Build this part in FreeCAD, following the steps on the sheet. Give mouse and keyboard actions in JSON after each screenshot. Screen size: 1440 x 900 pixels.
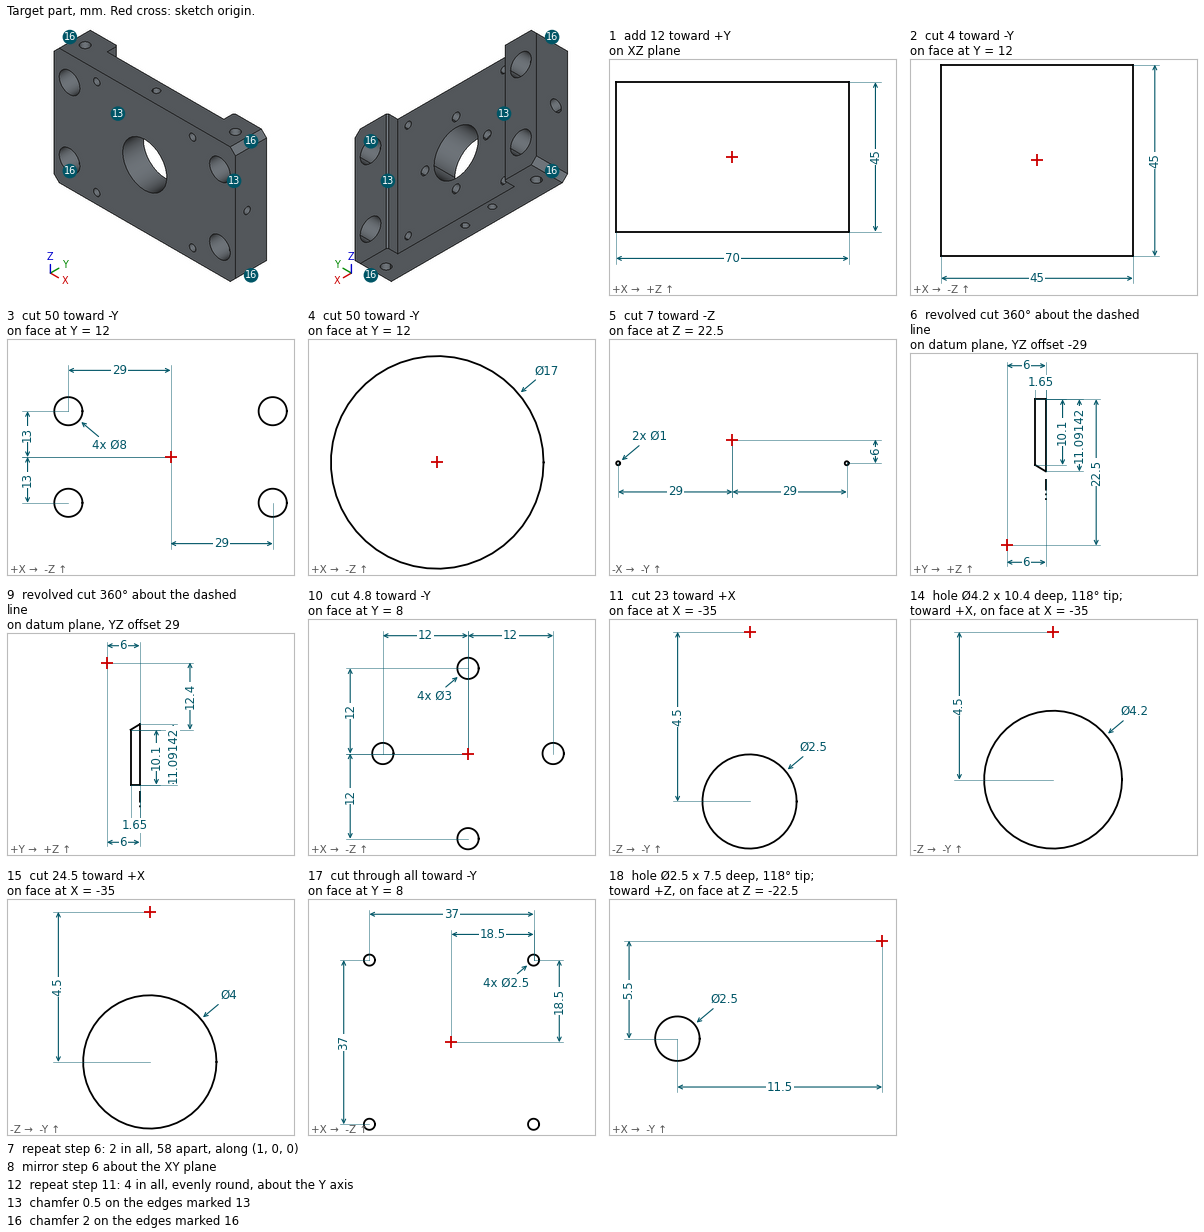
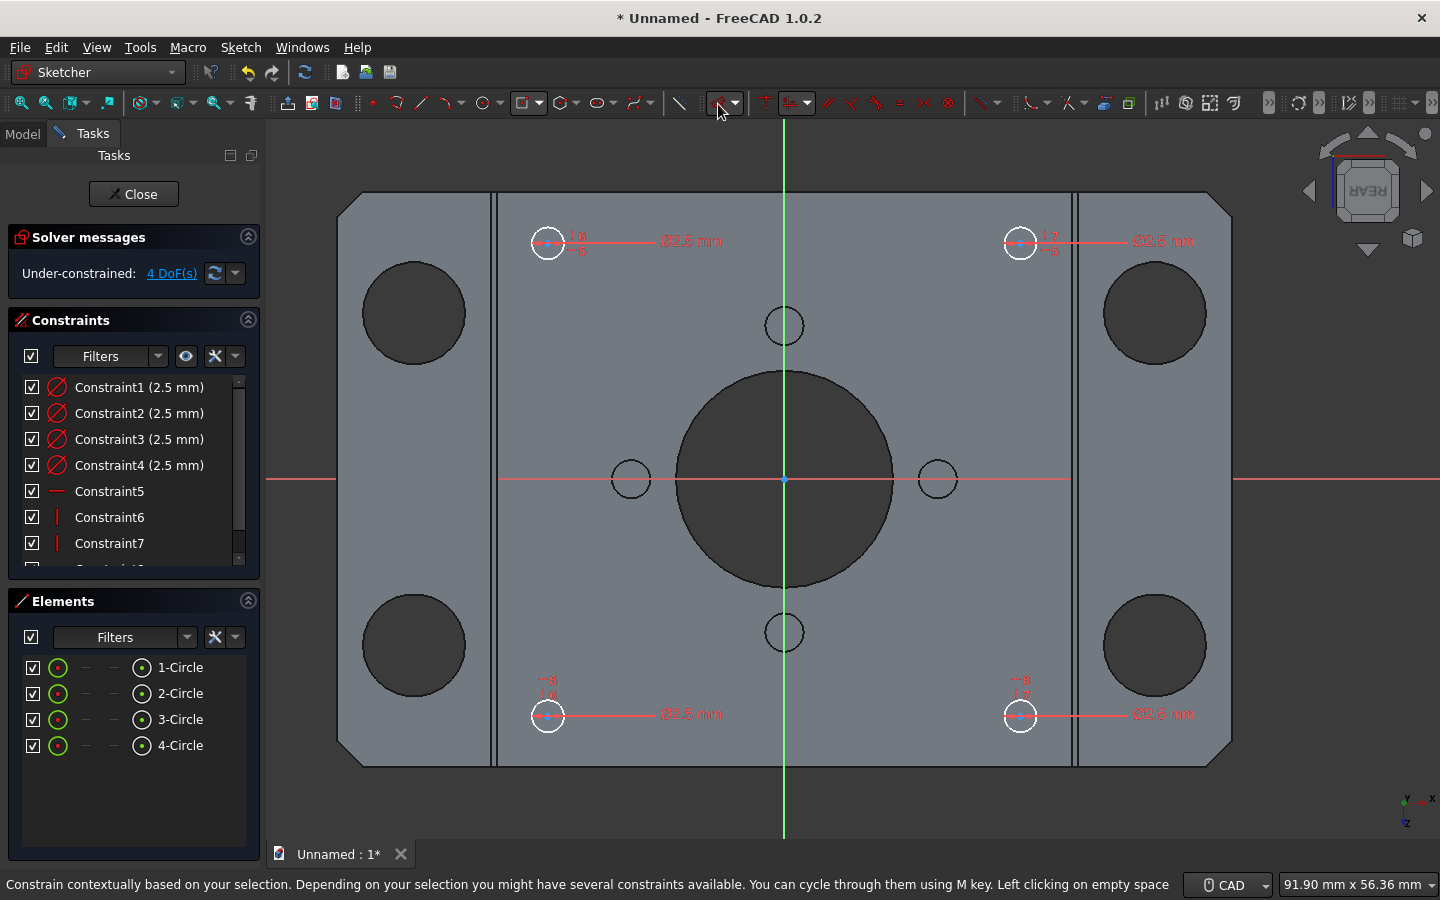
{"action": "left_click", "coordinate": [1021, 243]}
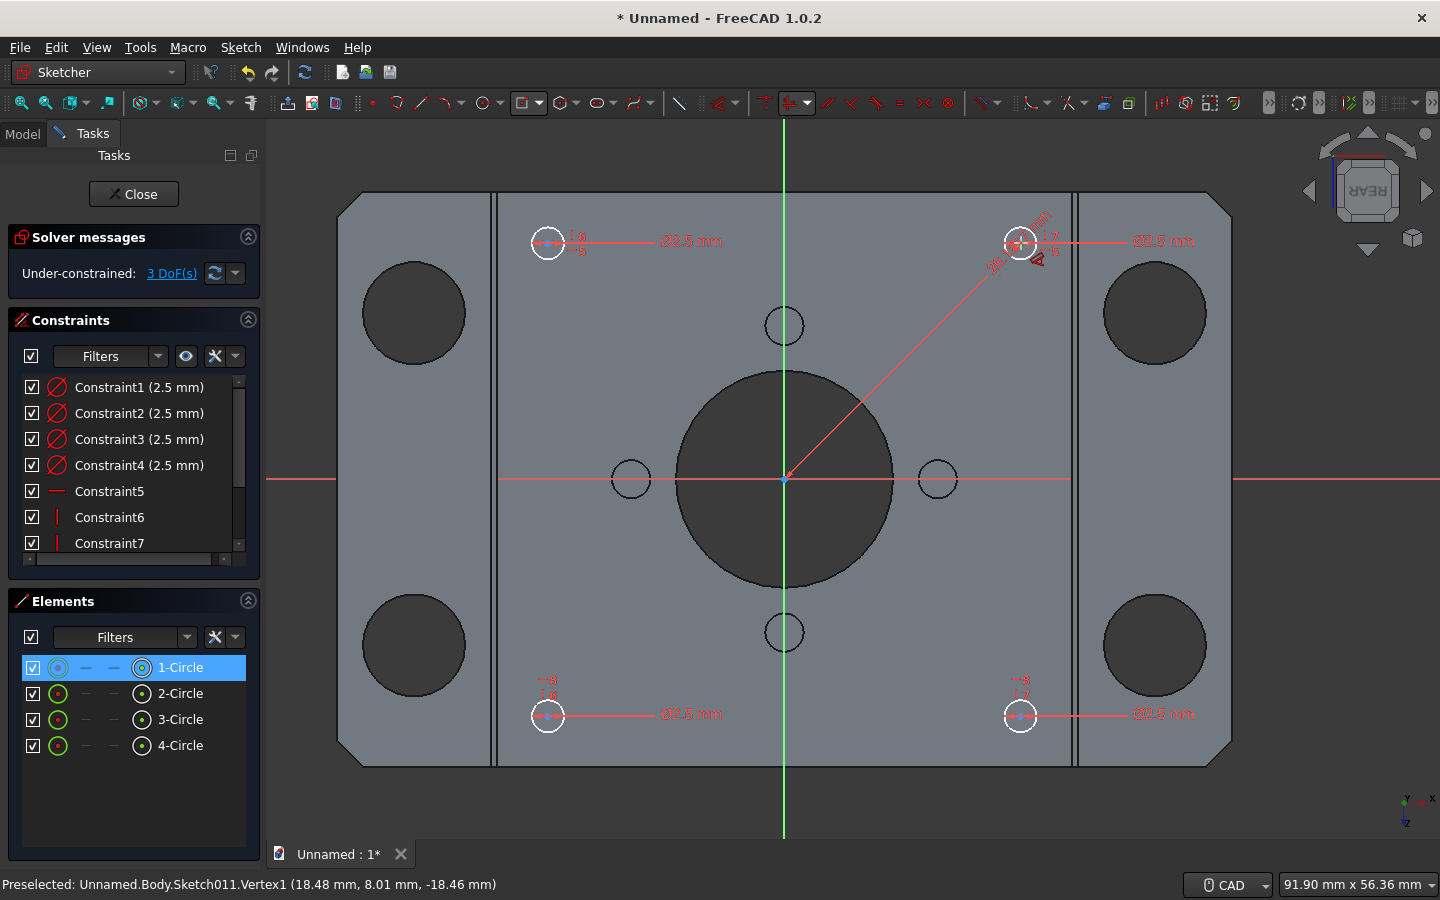
{"action": "left_click", "coordinate": [548, 243]}
{"action": "left_click", "coordinate": [676, 209]}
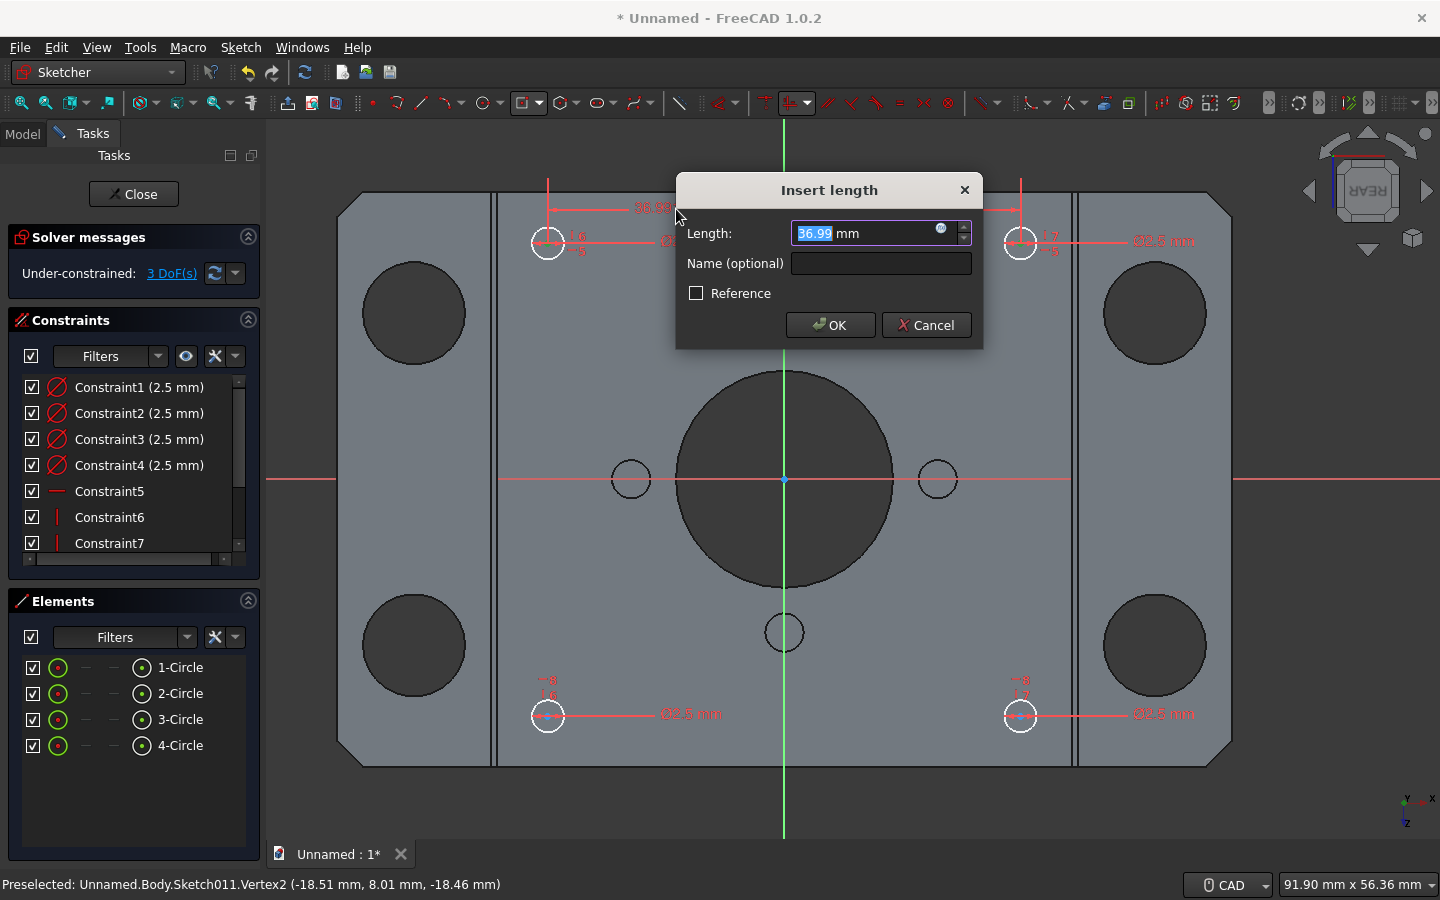
{"action": "type", "text": "37"}
{"action": "key", "text": "Return"}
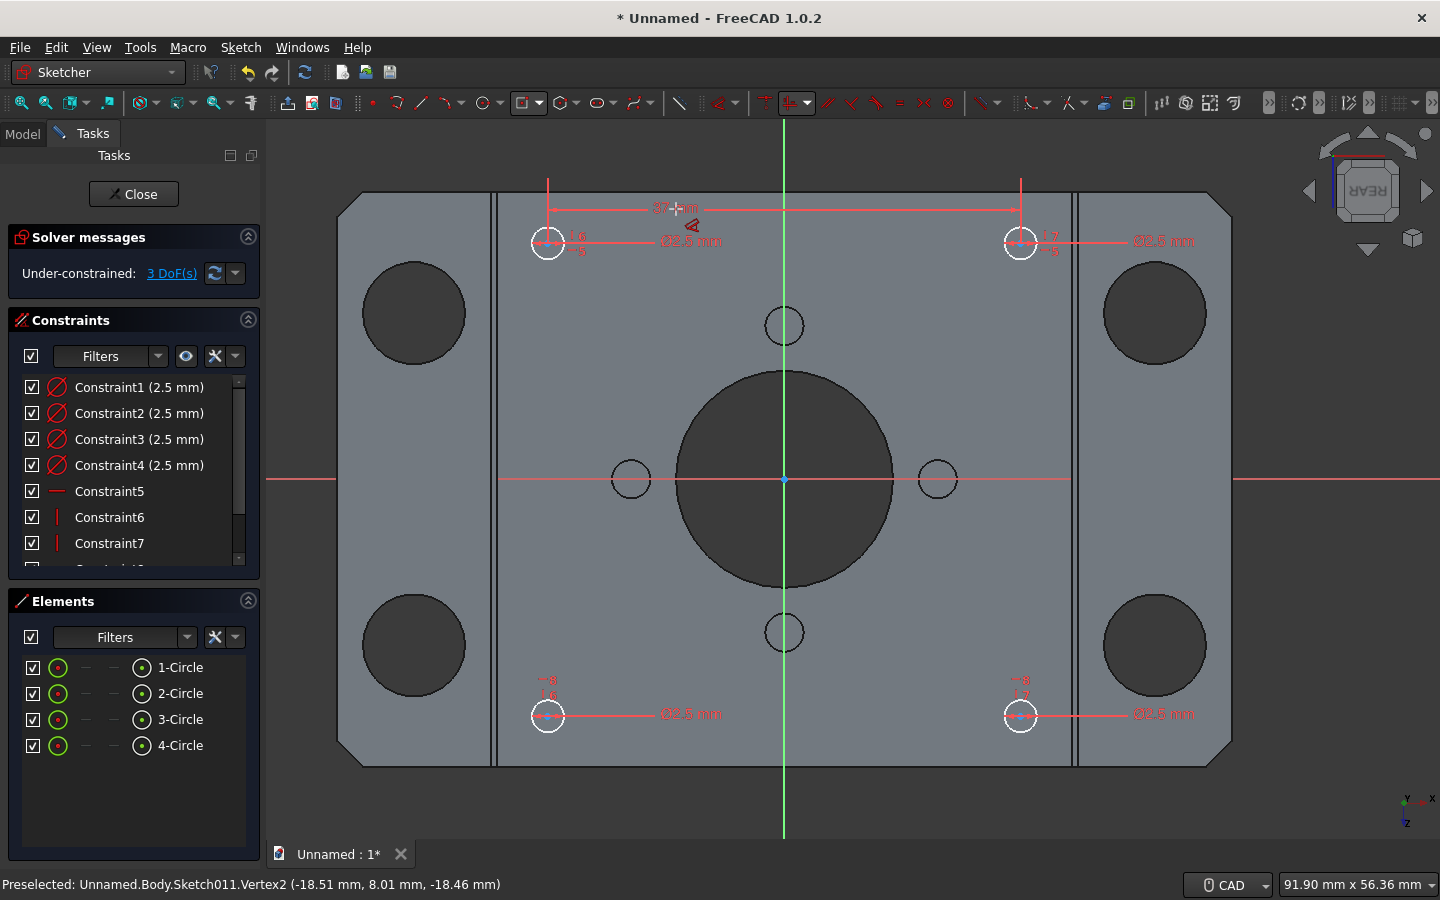
{"action": "left_click", "coordinate": [548, 243]}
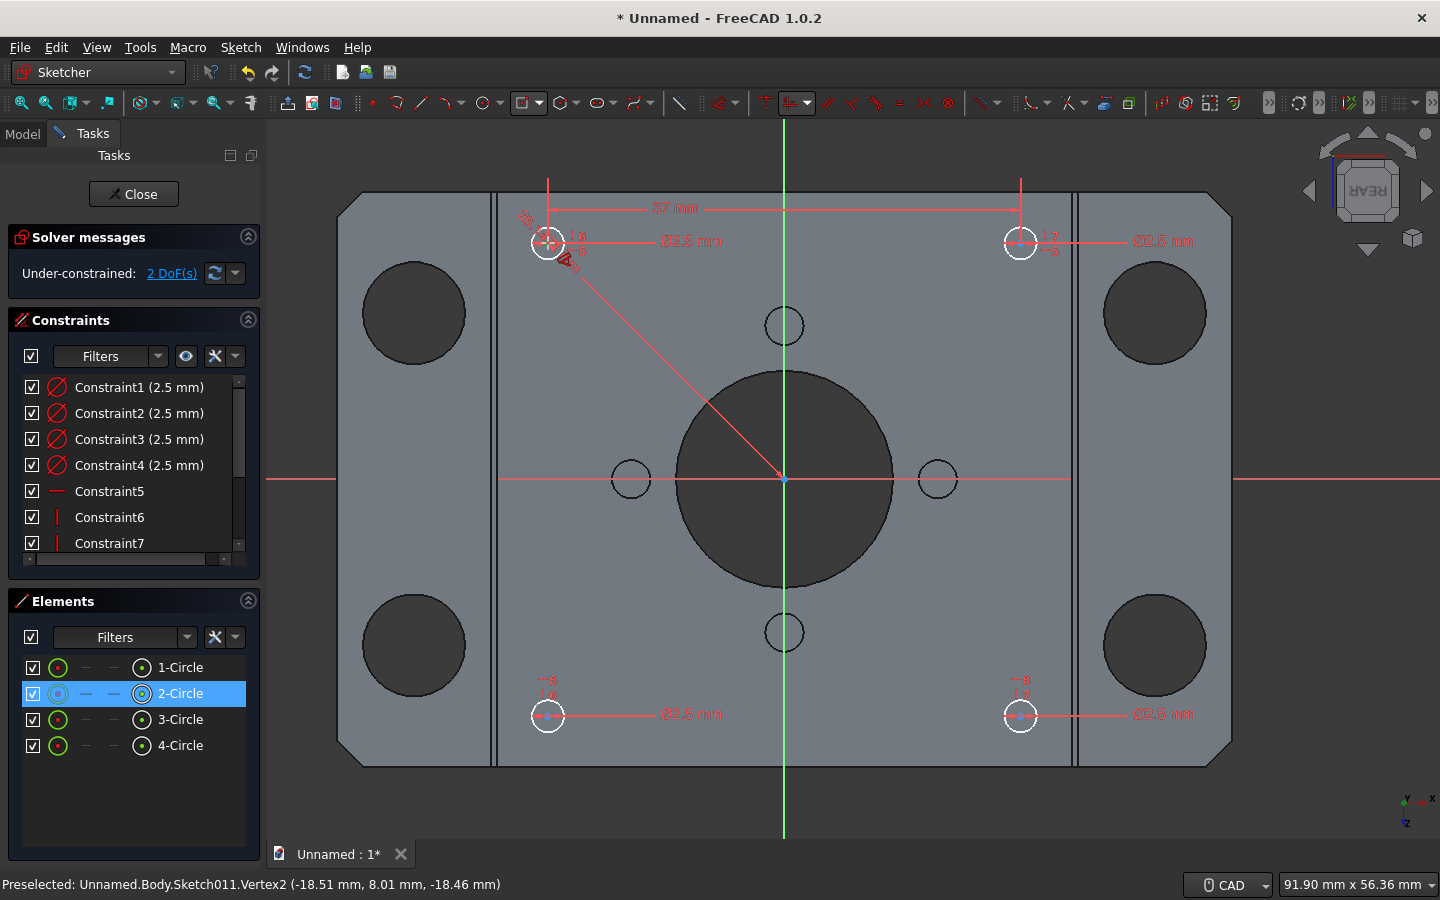
{"action": "left_click", "coordinate": [548, 716]}
{"action": "left_click", "coordinate": [514, 371]}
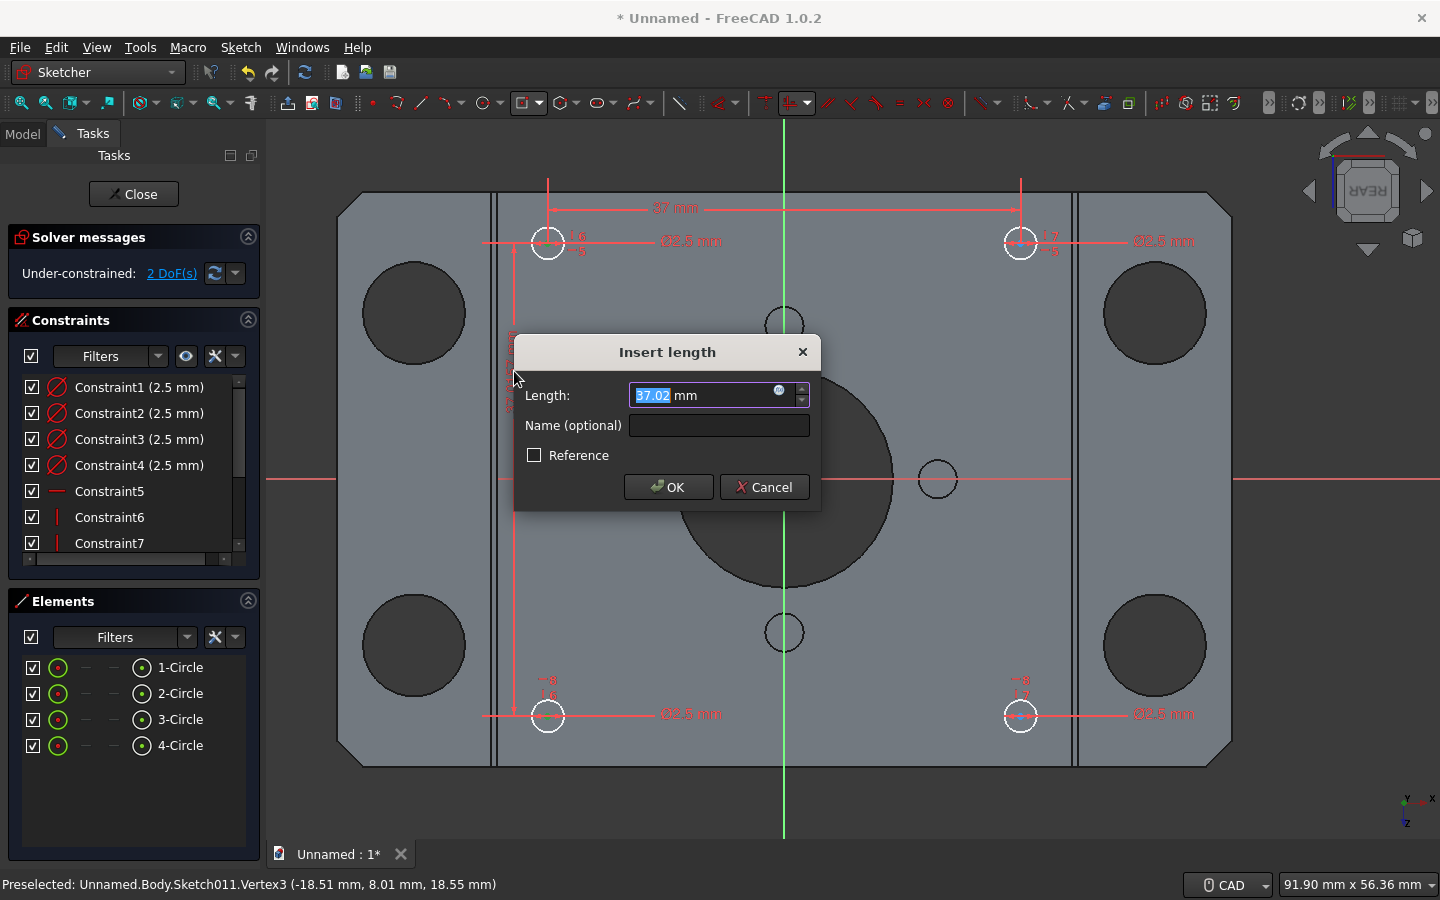
{"action": "type", "text": "37"}
{"action": "key", "text": "Return"}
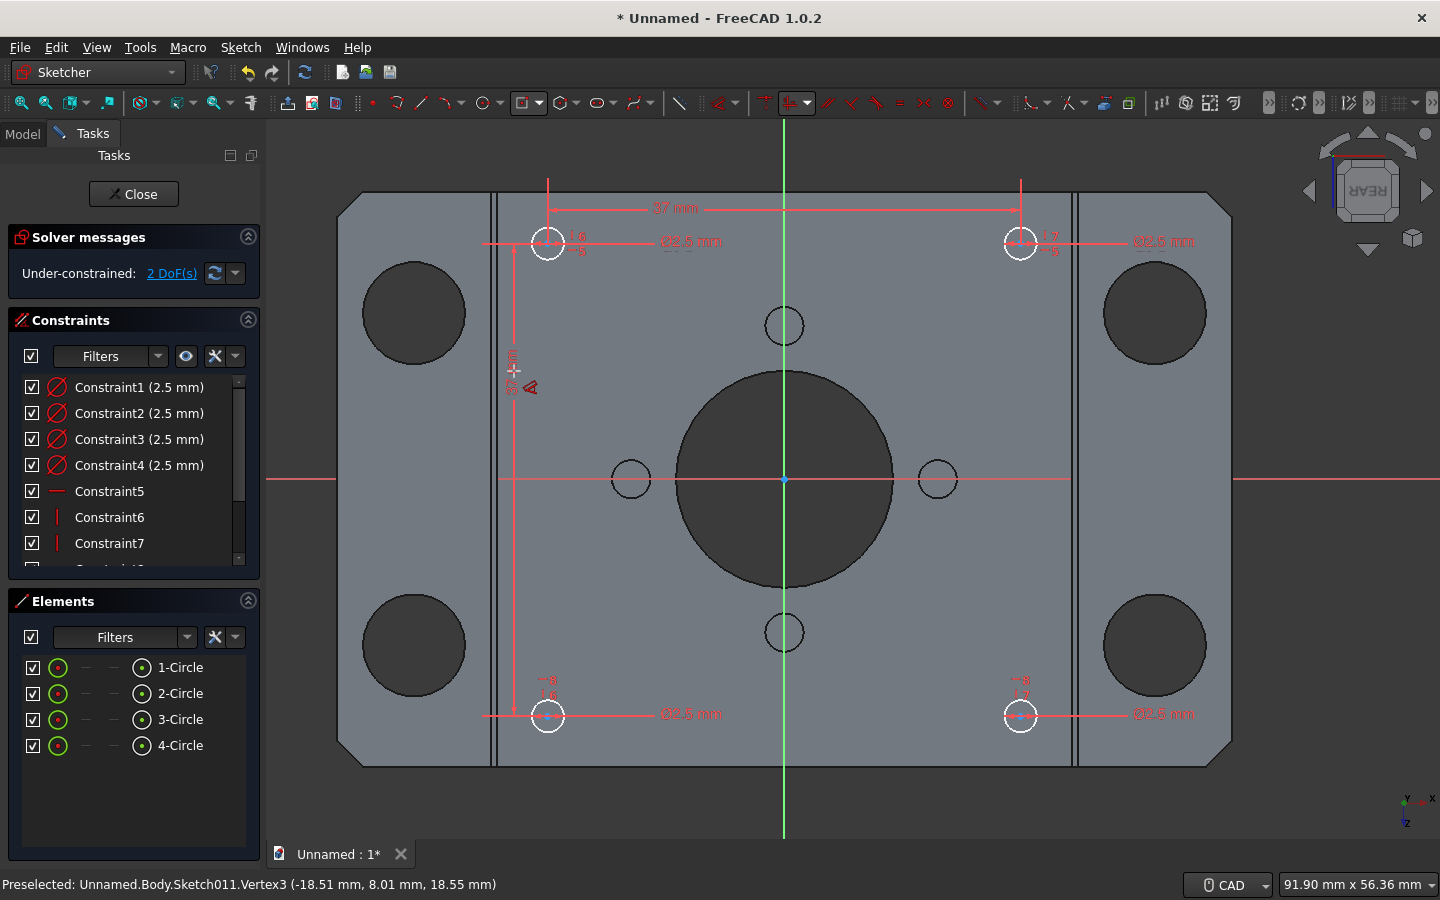
{"action": "left_click", "coordinate": [1021, 244]}
{"action": "left_click", "coordinate": [903, 210]}